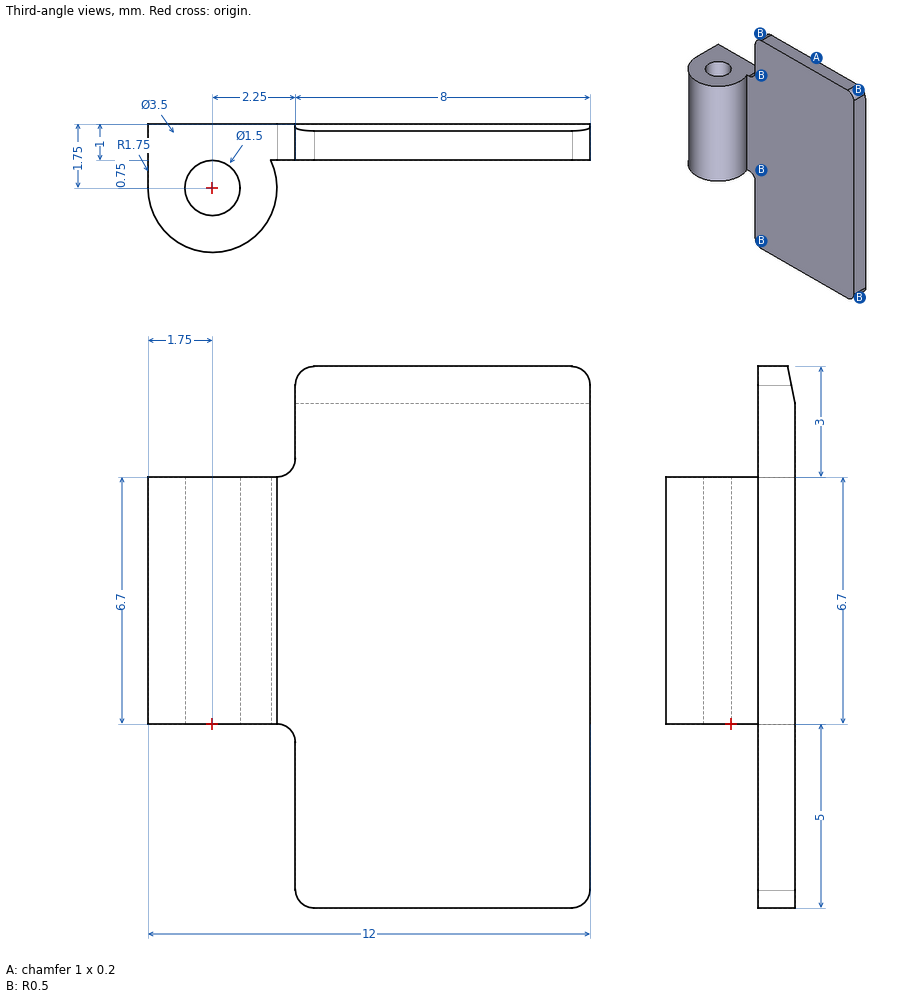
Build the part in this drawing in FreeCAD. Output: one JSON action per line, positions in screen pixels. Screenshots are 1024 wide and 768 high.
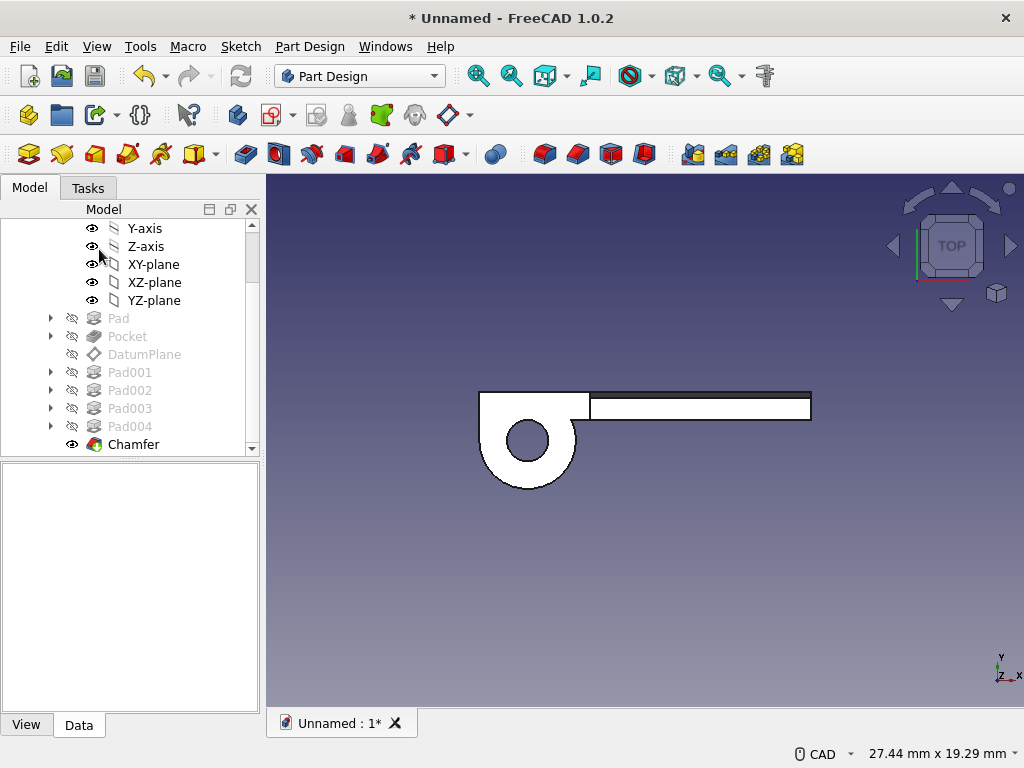
{"action": "key", "text": "v f"}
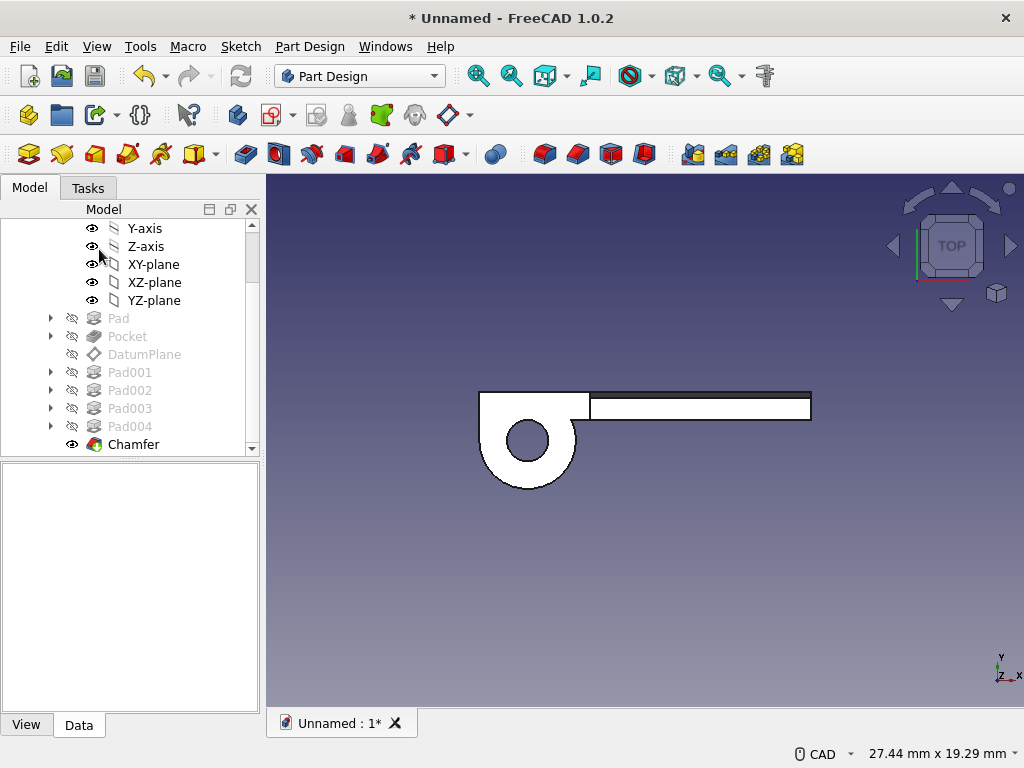
{"action": "left_click", "coordinate": [811, 408]}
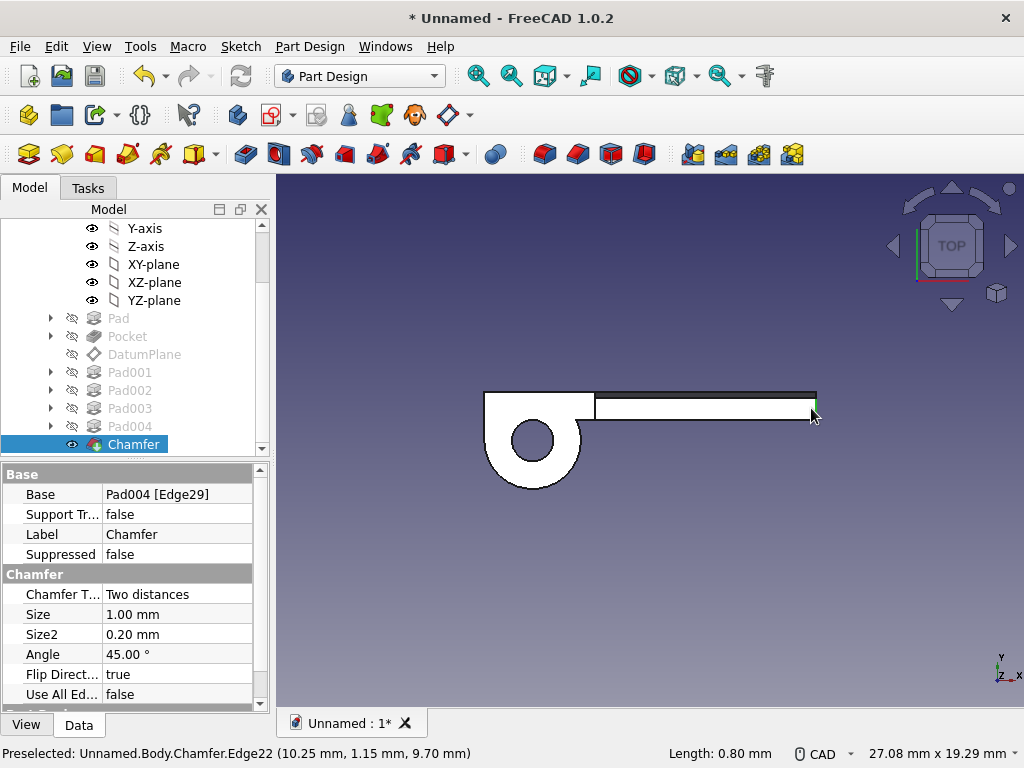
{"action": "left_click", "coordinate": [595, 408], "text": "ctrl"}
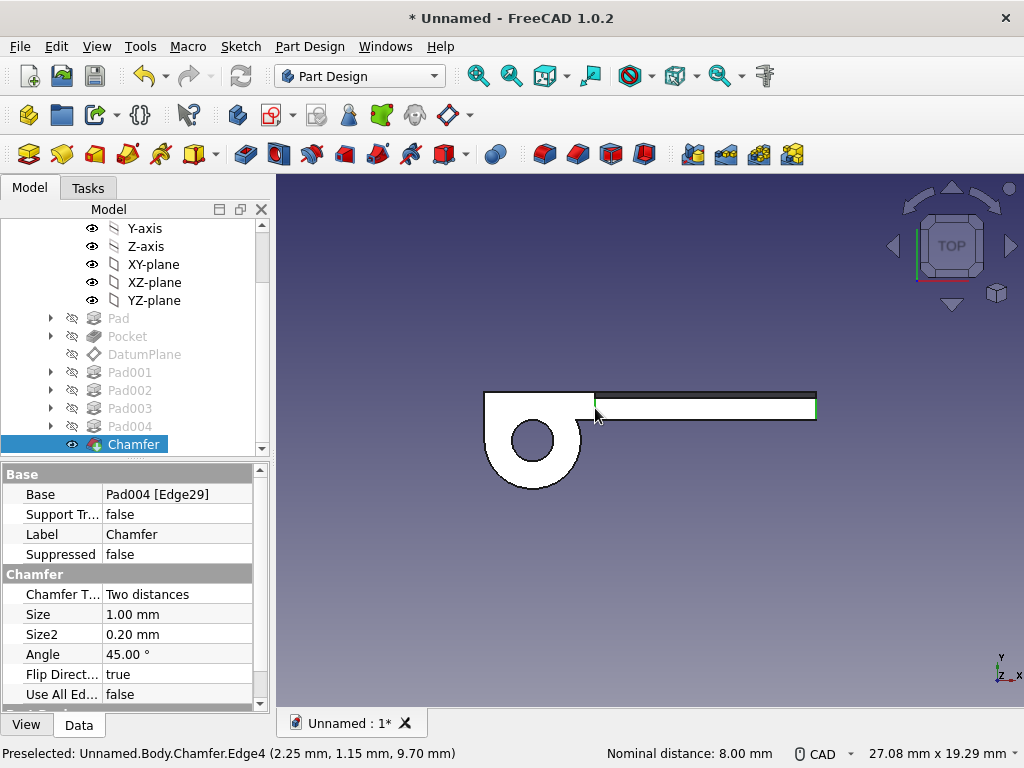
{"action": "key", "text": "0"}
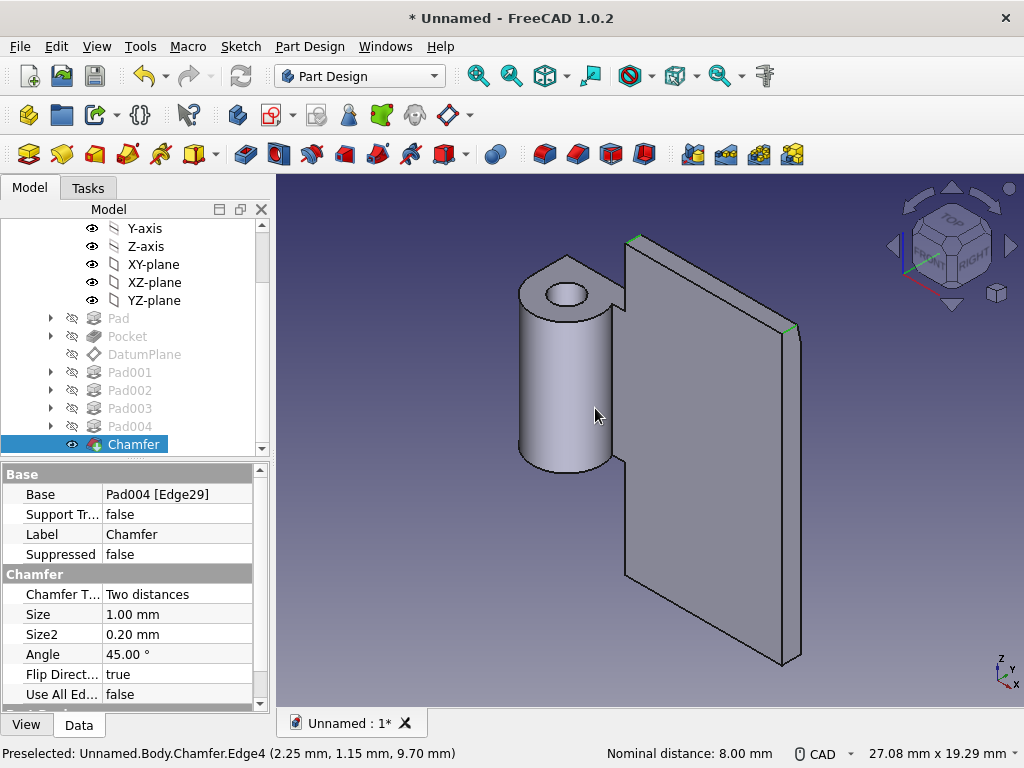
{"action": "key", "text": "2"}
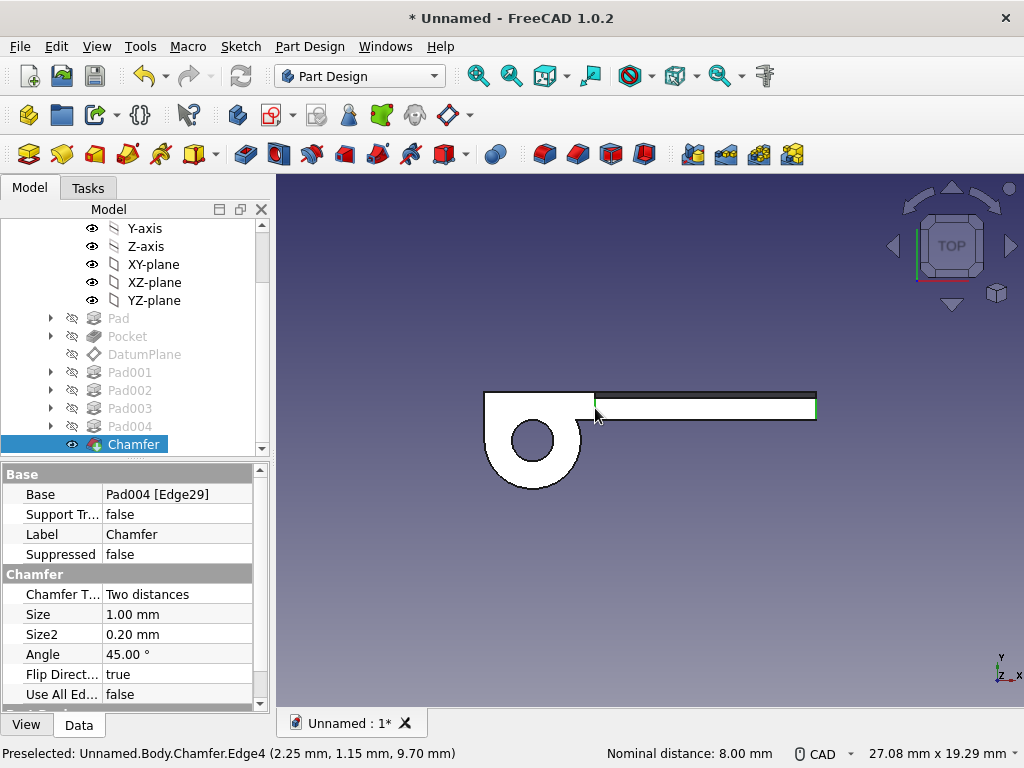
{"action": "left_click", "coordinate": [479, 76]}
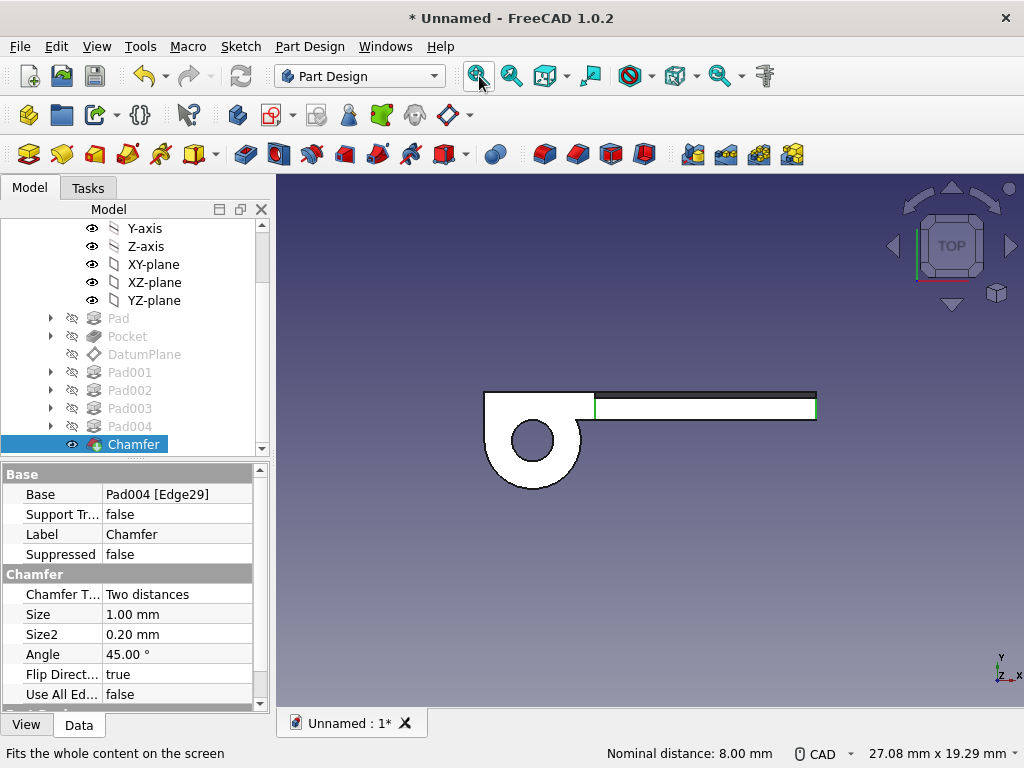
{"action": "key", "text": "1"}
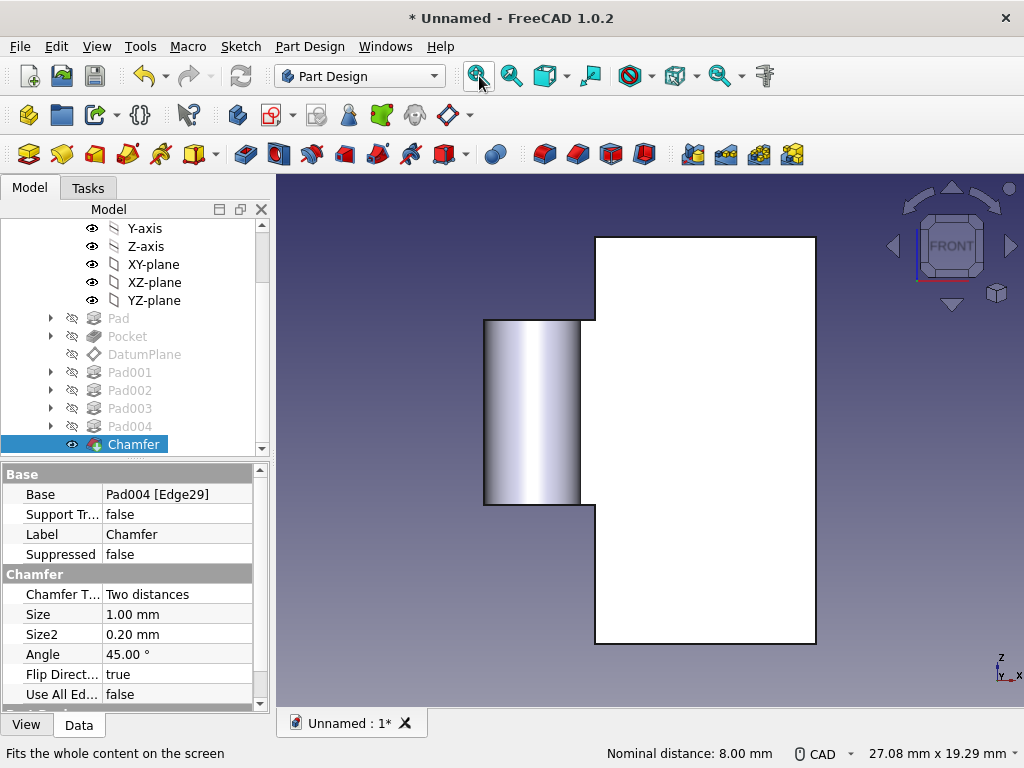
{"action": "key", "text": "3"}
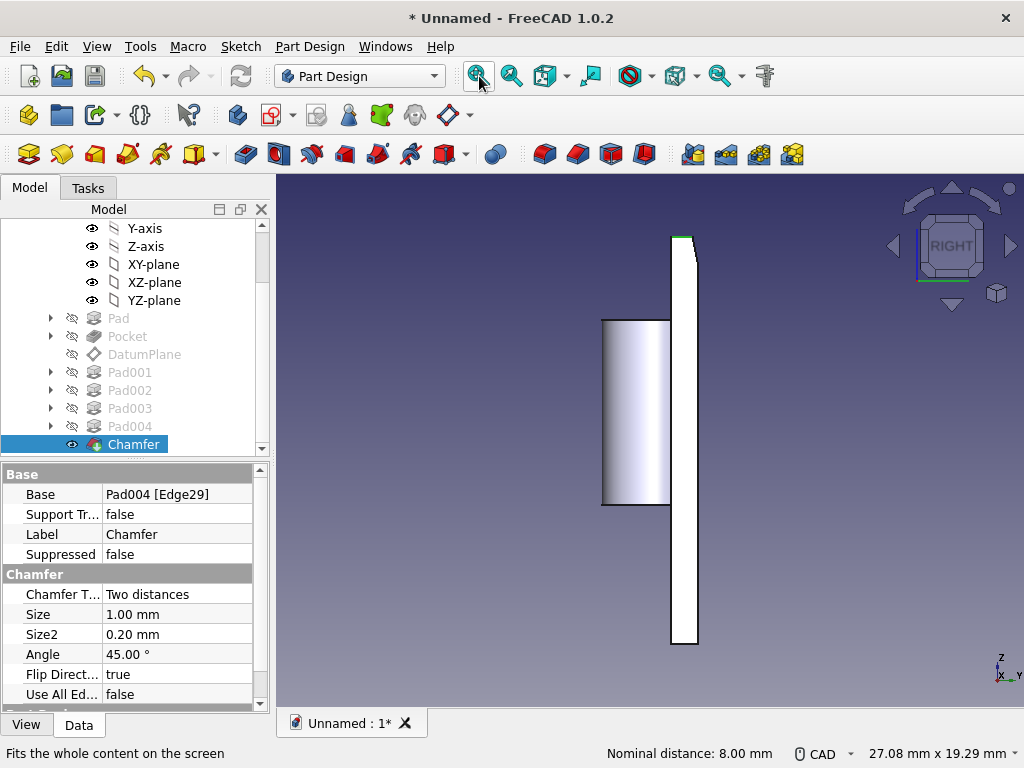
{"action": "left_click", "coordinate": [684, 643], "text": "ctrl"}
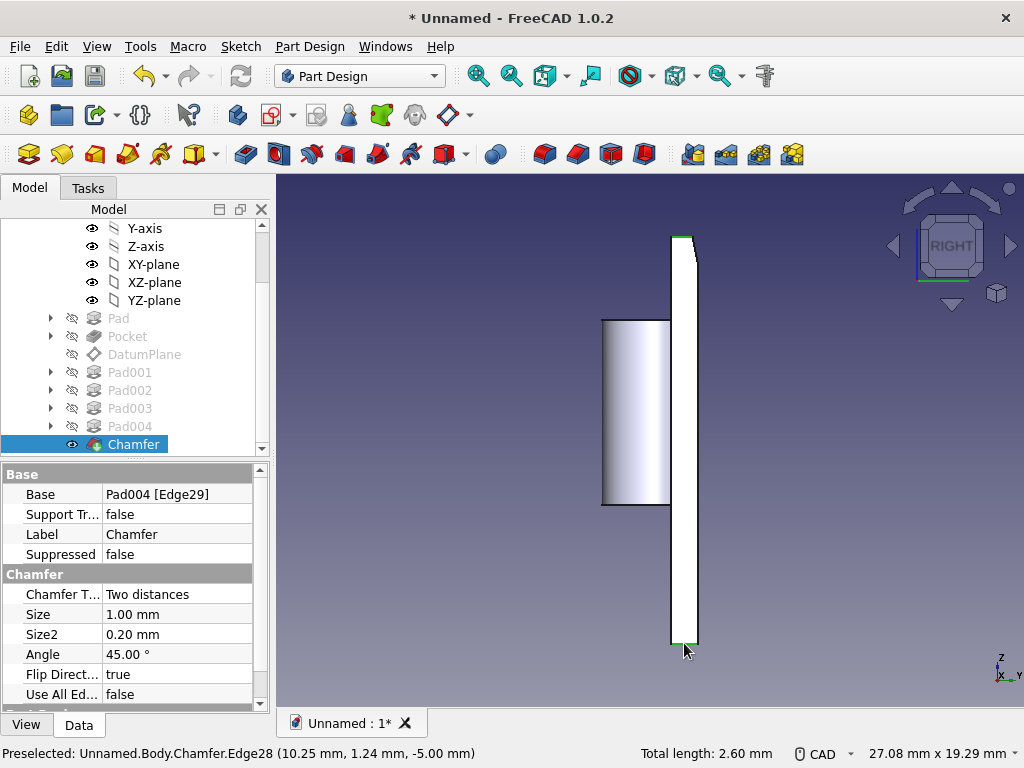
{"action": "key", "text": "5"}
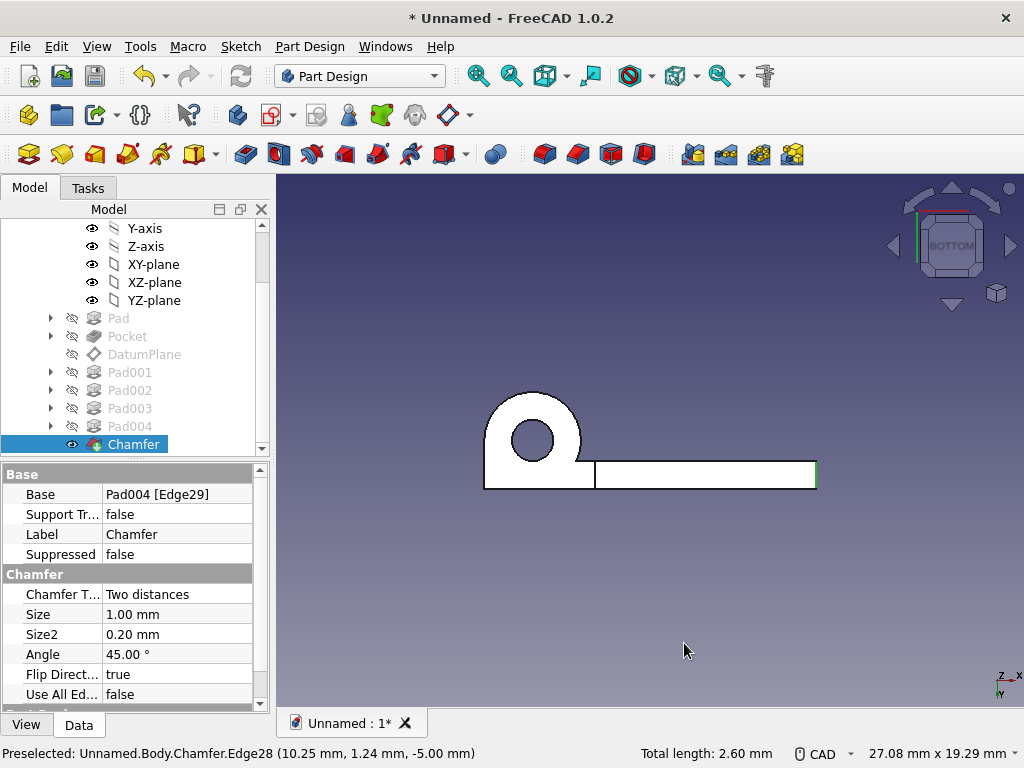
{"action": "left_click", "coordinate": [479, 76]}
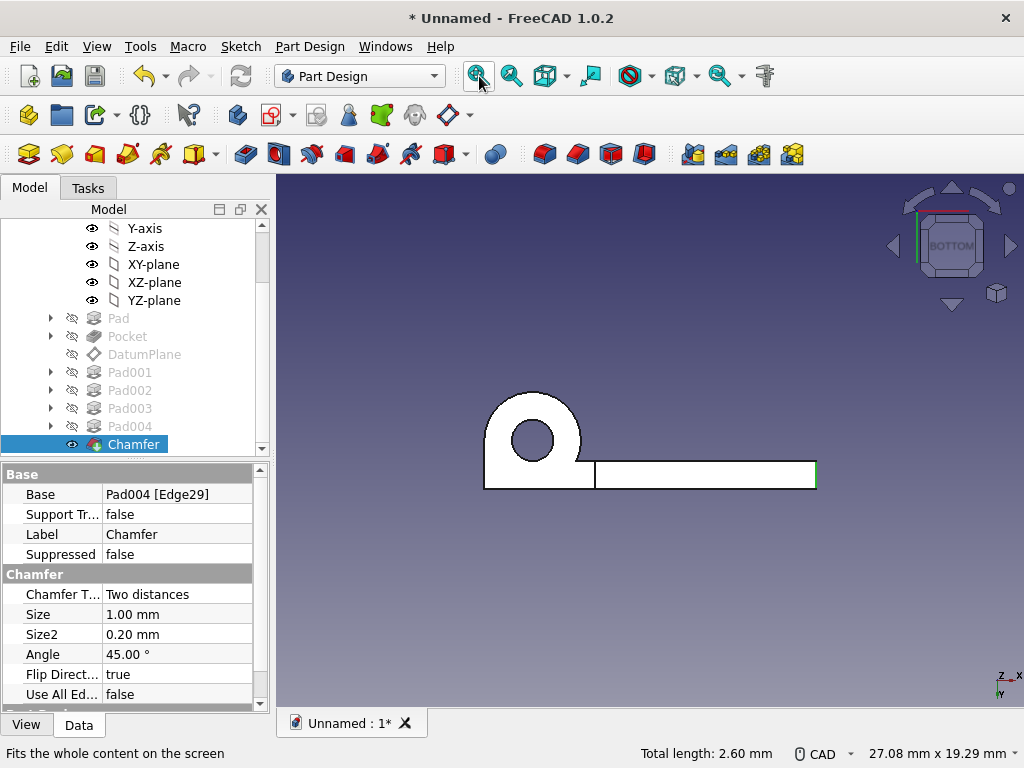
{"action": "left_click", "coordinate": [595, 474], "text": "ctrl"}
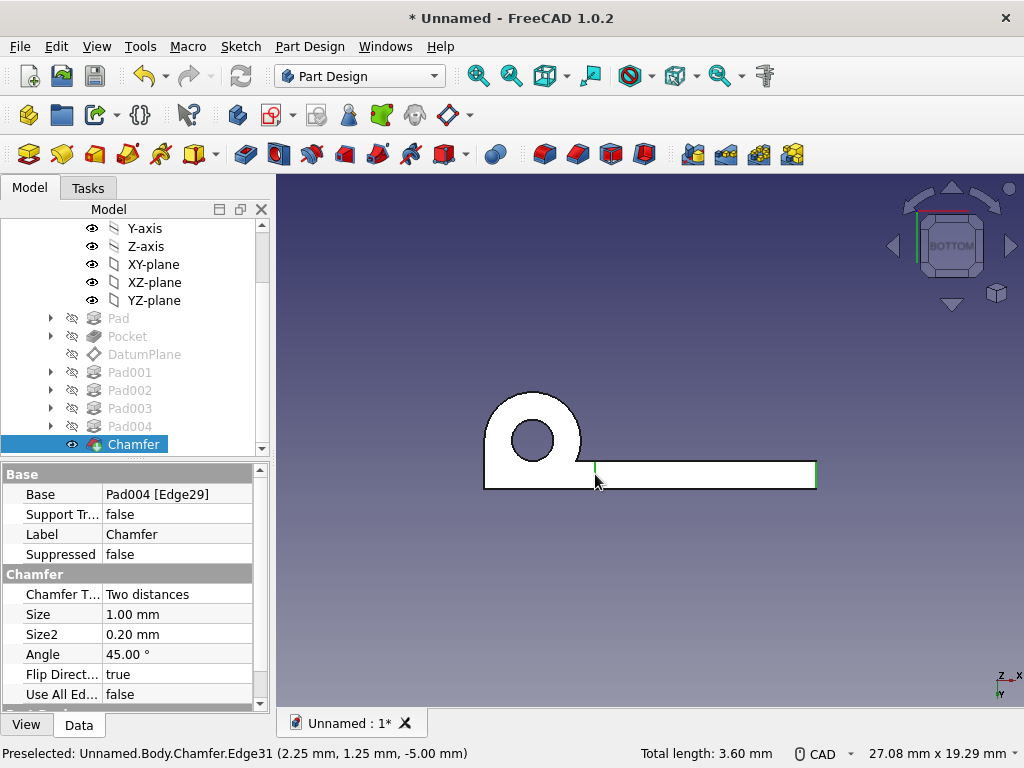
{"action": "key", "text": "4"}